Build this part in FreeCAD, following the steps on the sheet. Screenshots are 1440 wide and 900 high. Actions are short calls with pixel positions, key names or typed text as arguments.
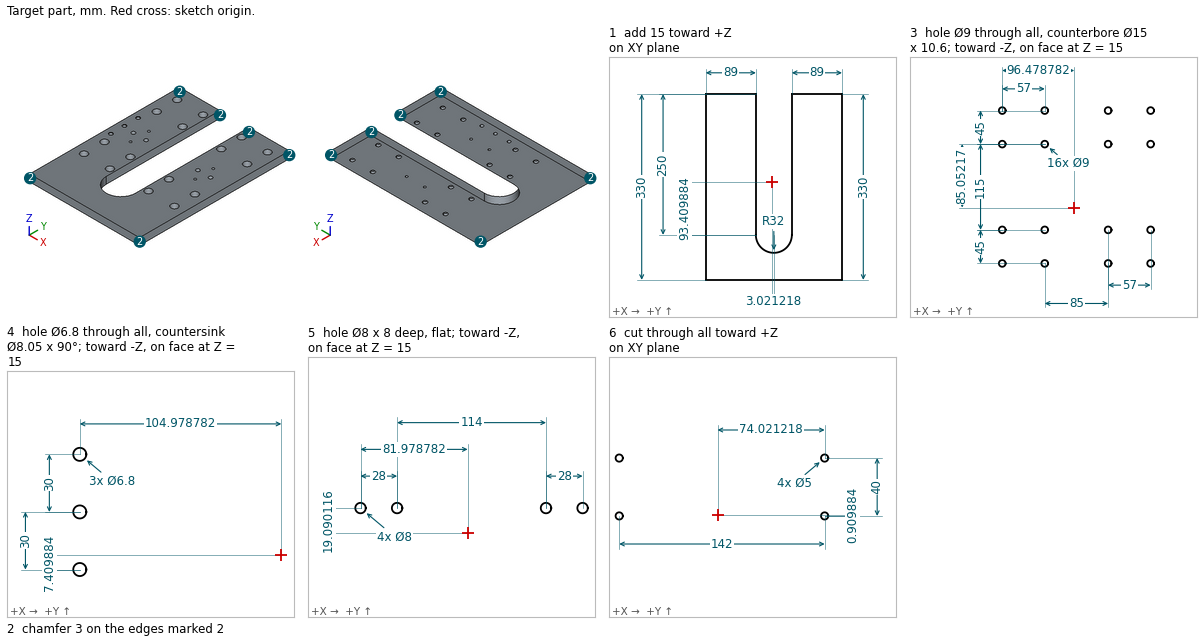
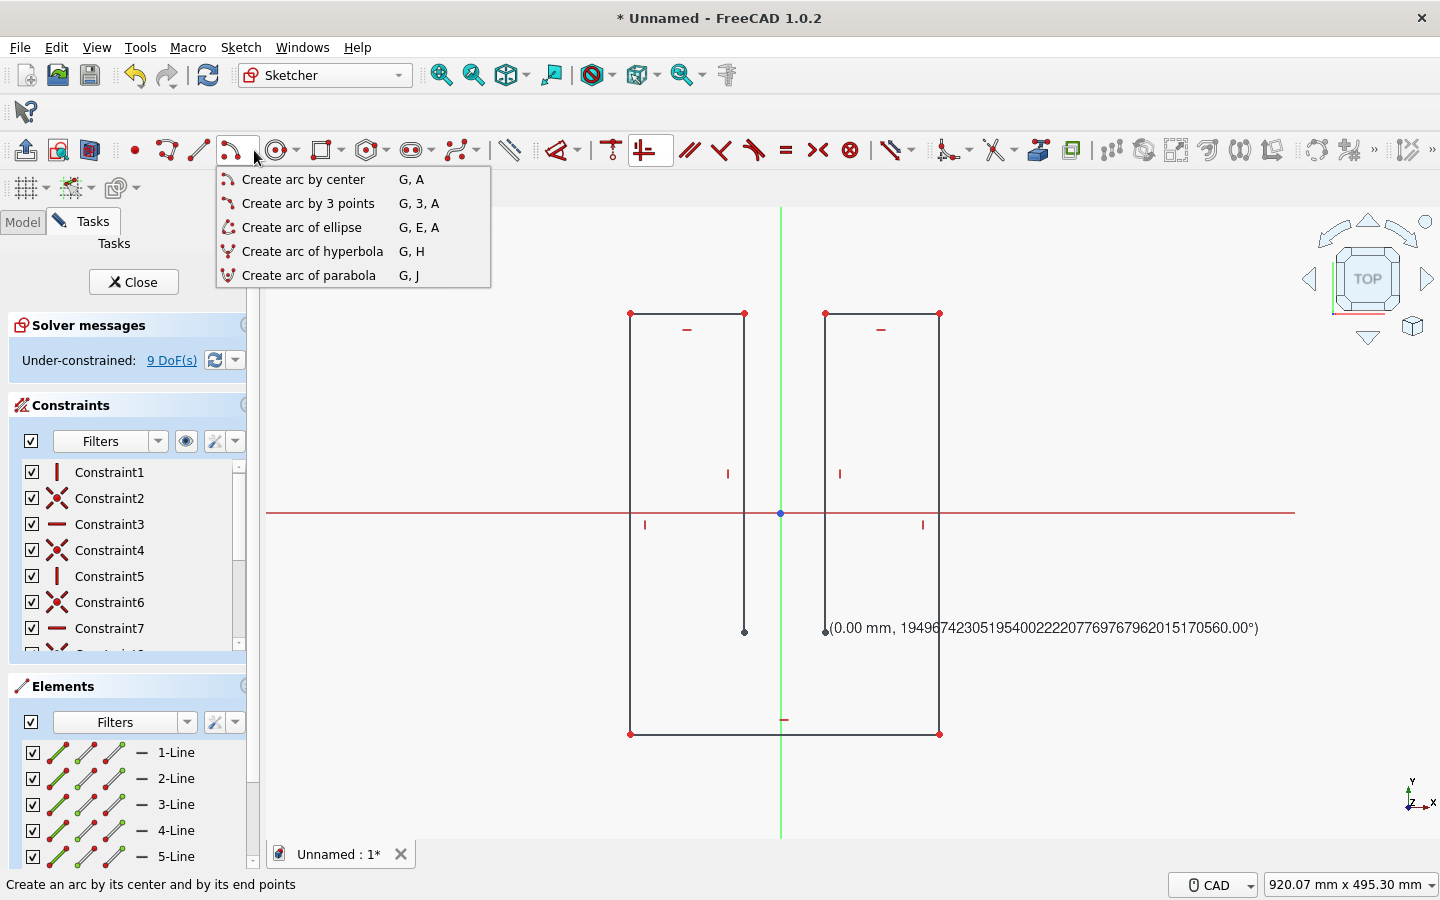
click(354, 203)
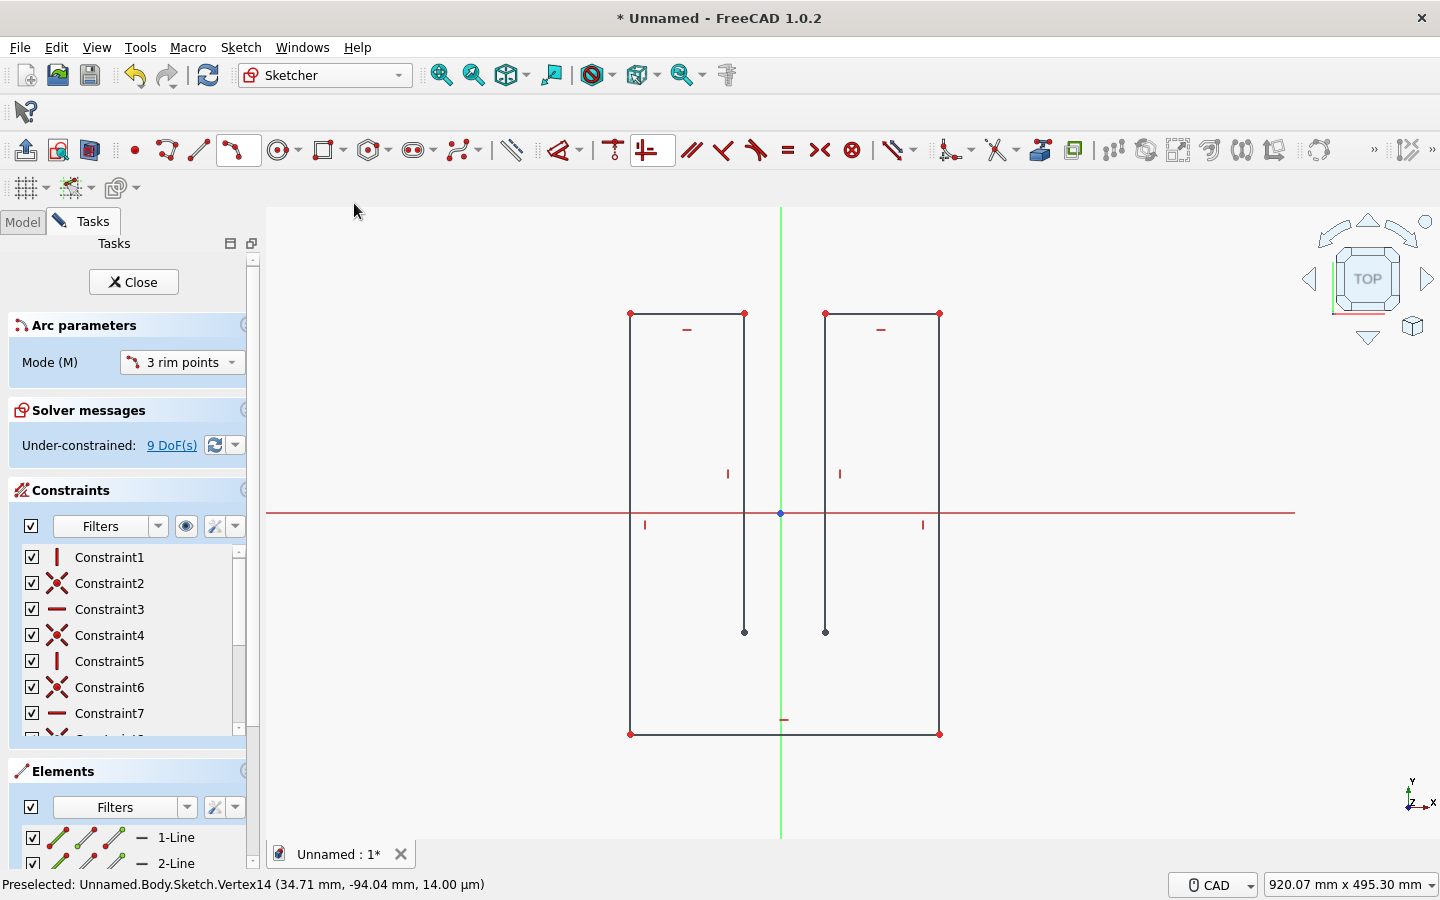
click(825, 633)
click(744, 633)
click(797, 671)
key(Escape)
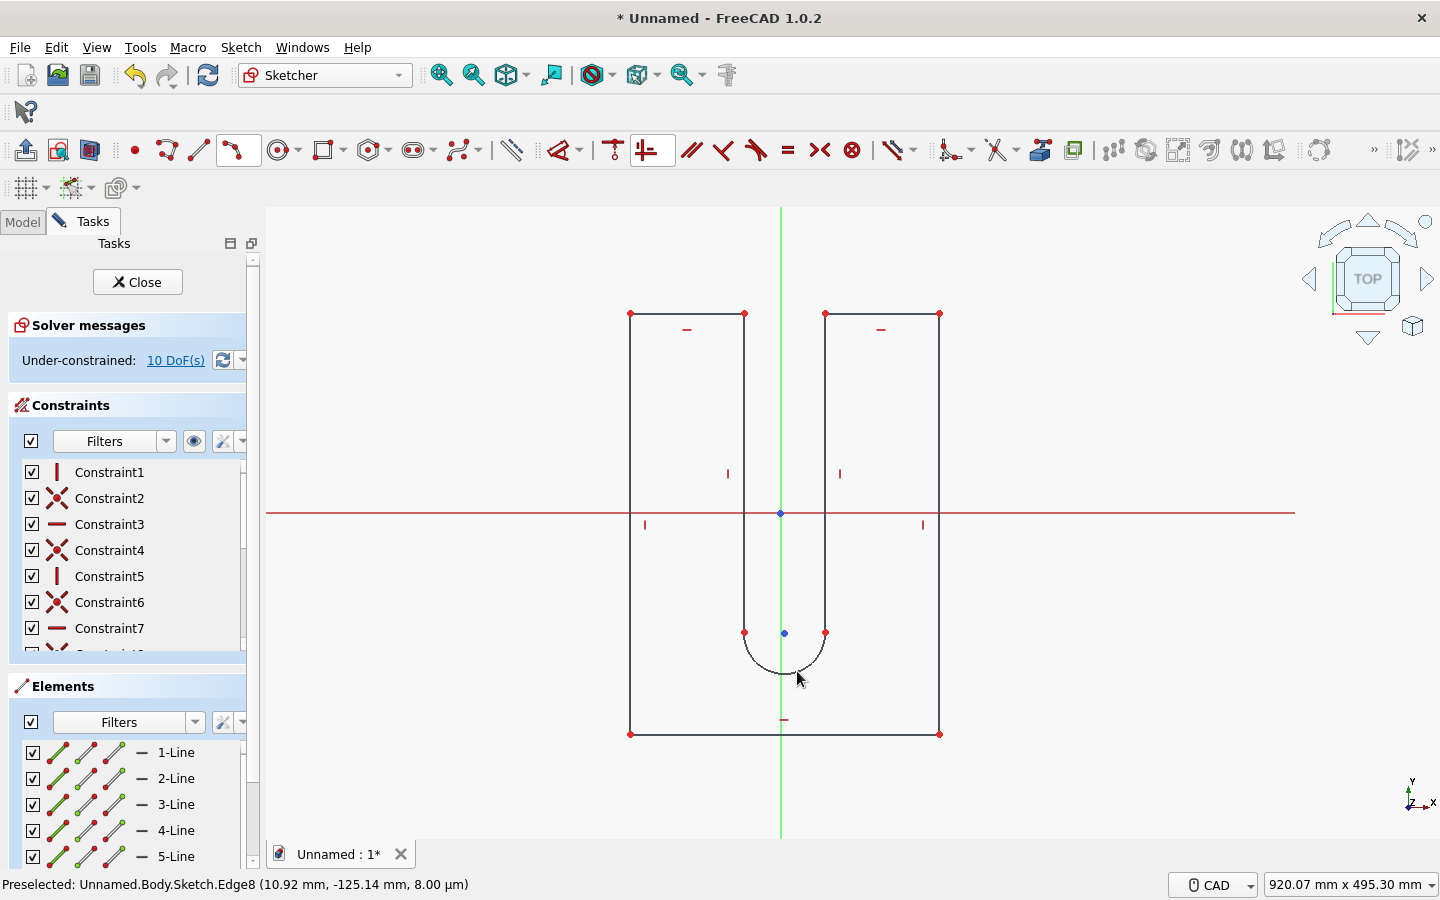
click(744, 537)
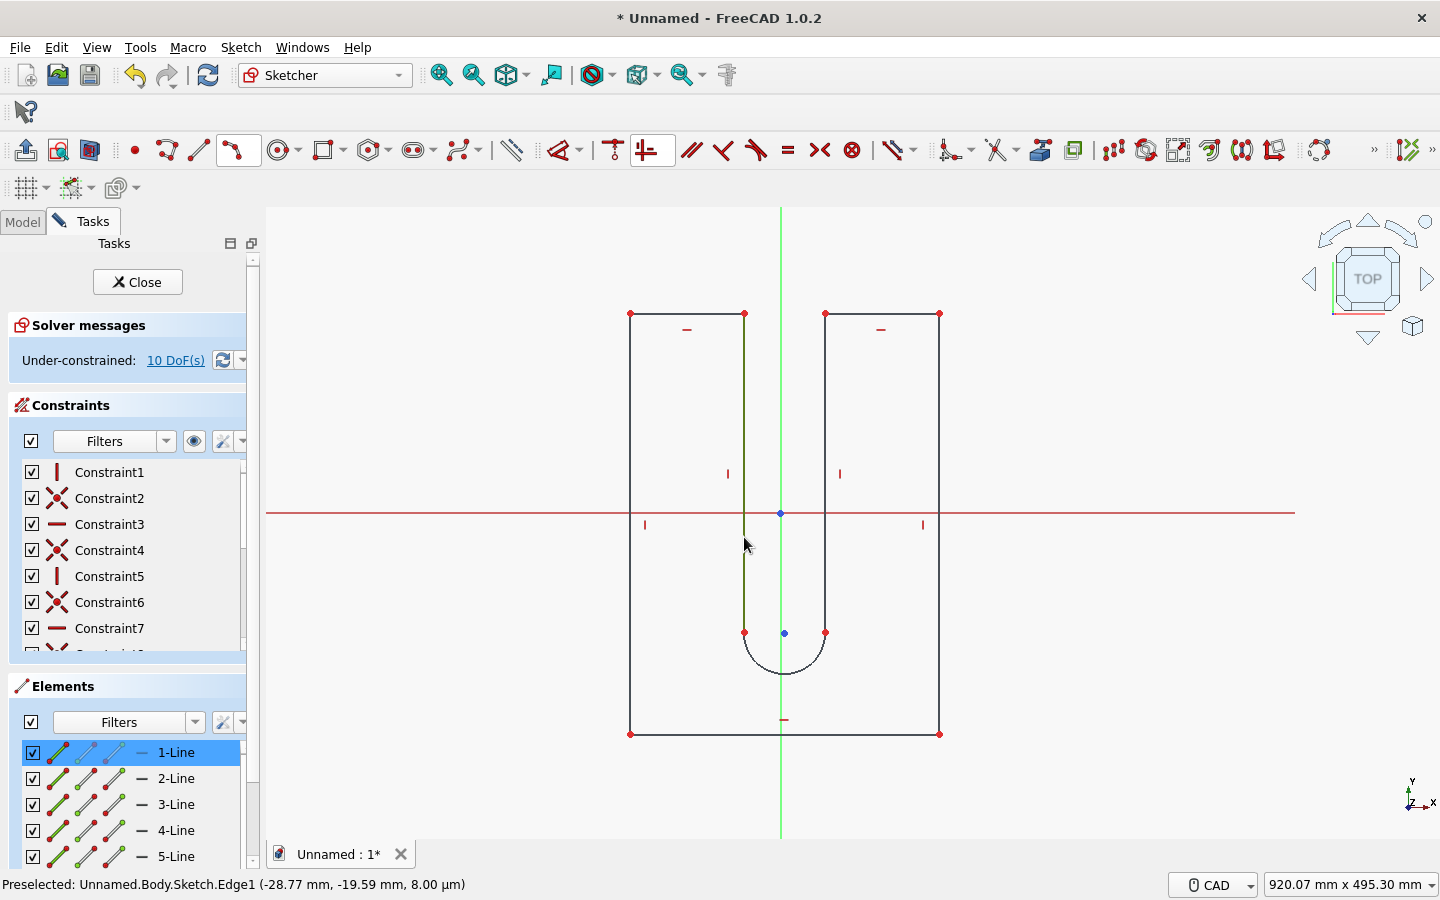
click(761, 666)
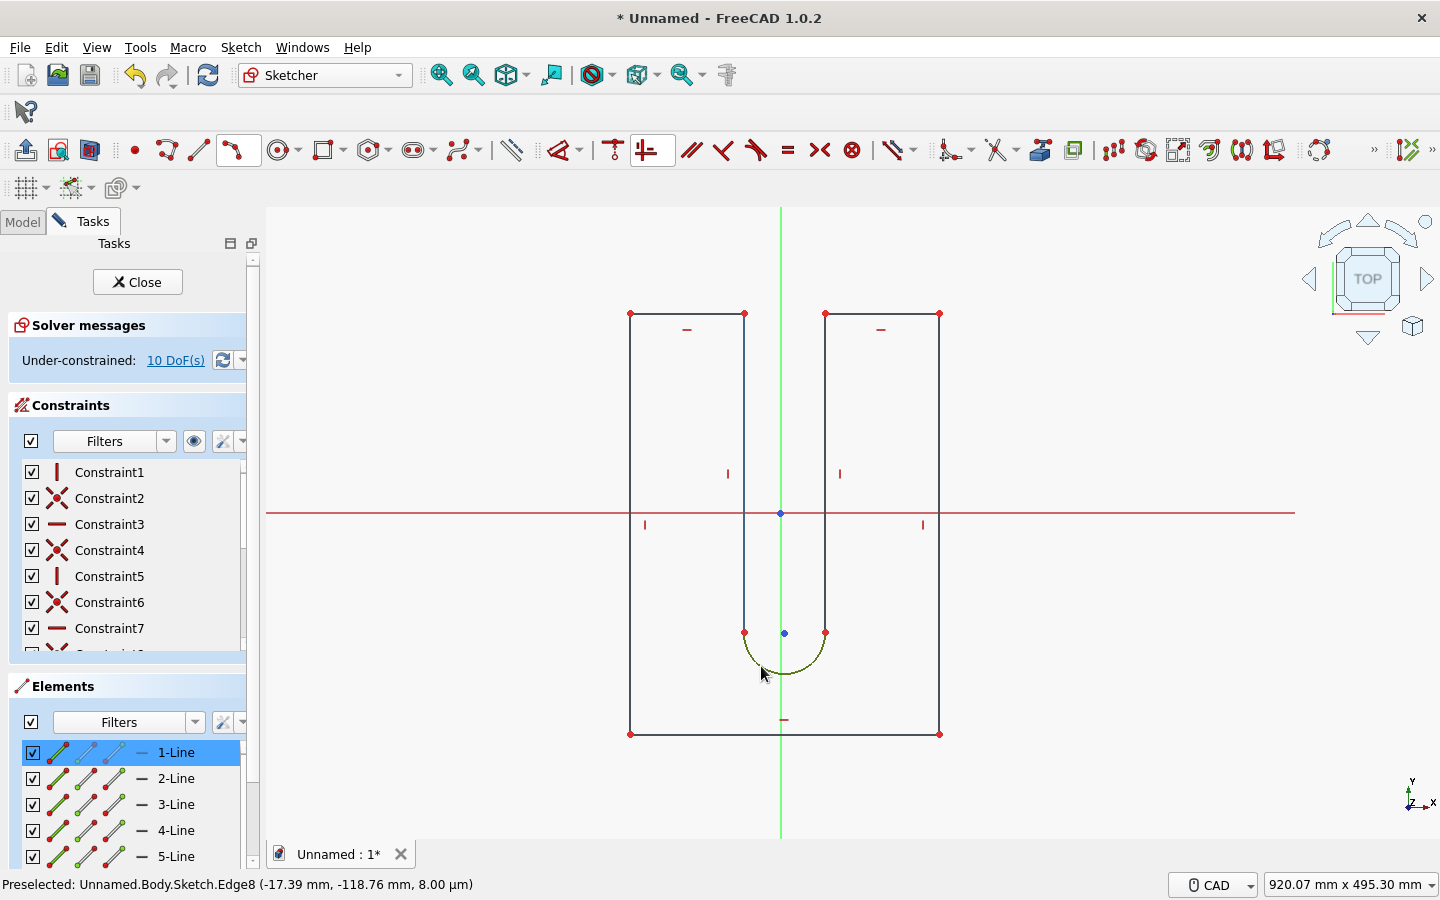
click(756, 150)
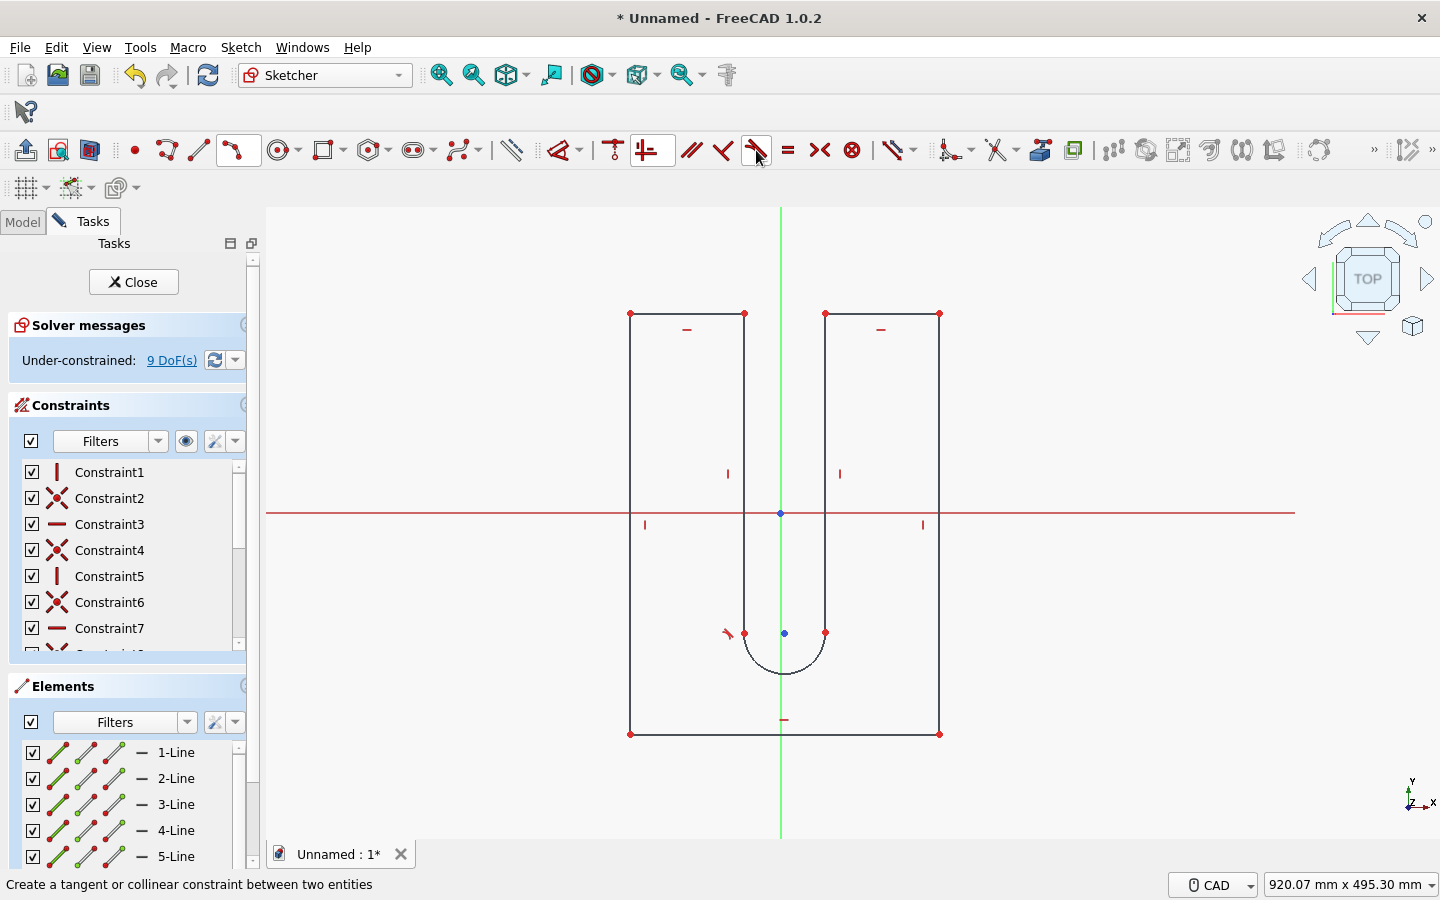
click(825, 410)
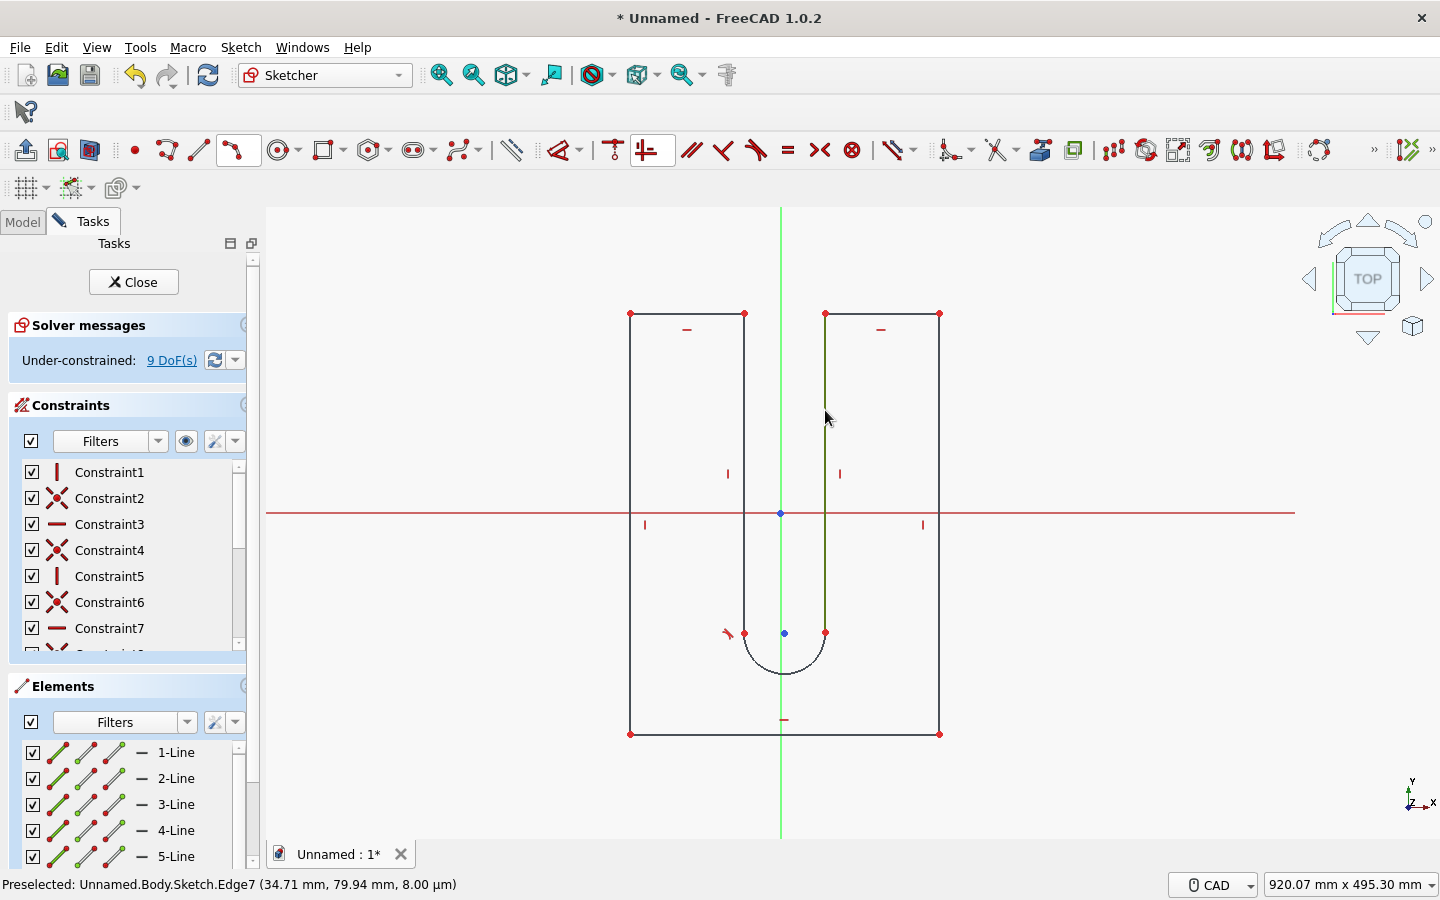
click(761, 666)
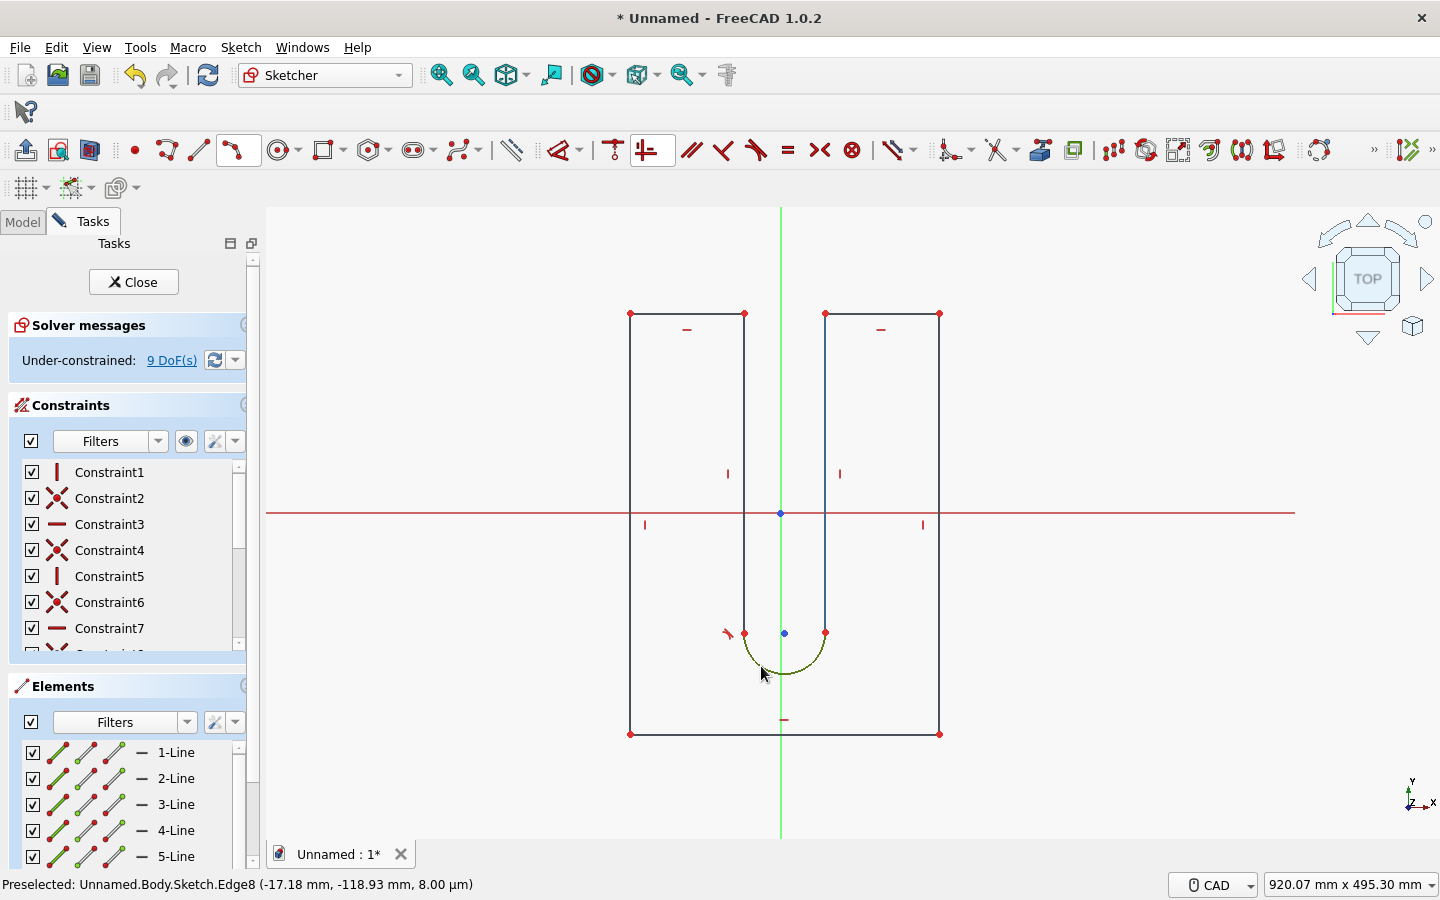
click(756, 150)